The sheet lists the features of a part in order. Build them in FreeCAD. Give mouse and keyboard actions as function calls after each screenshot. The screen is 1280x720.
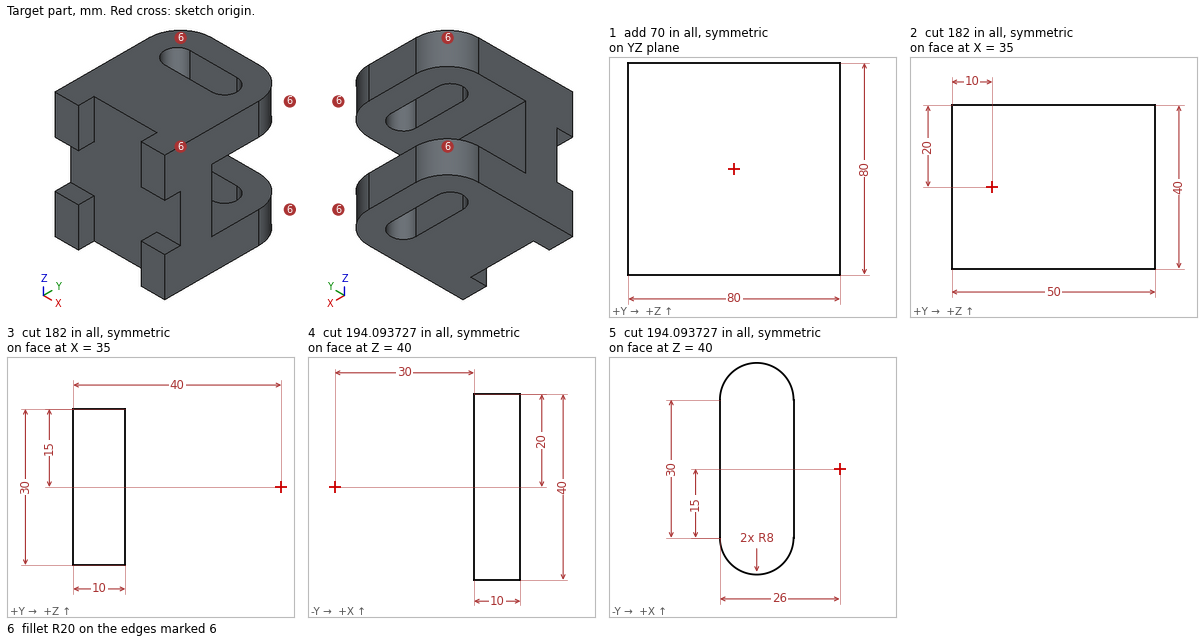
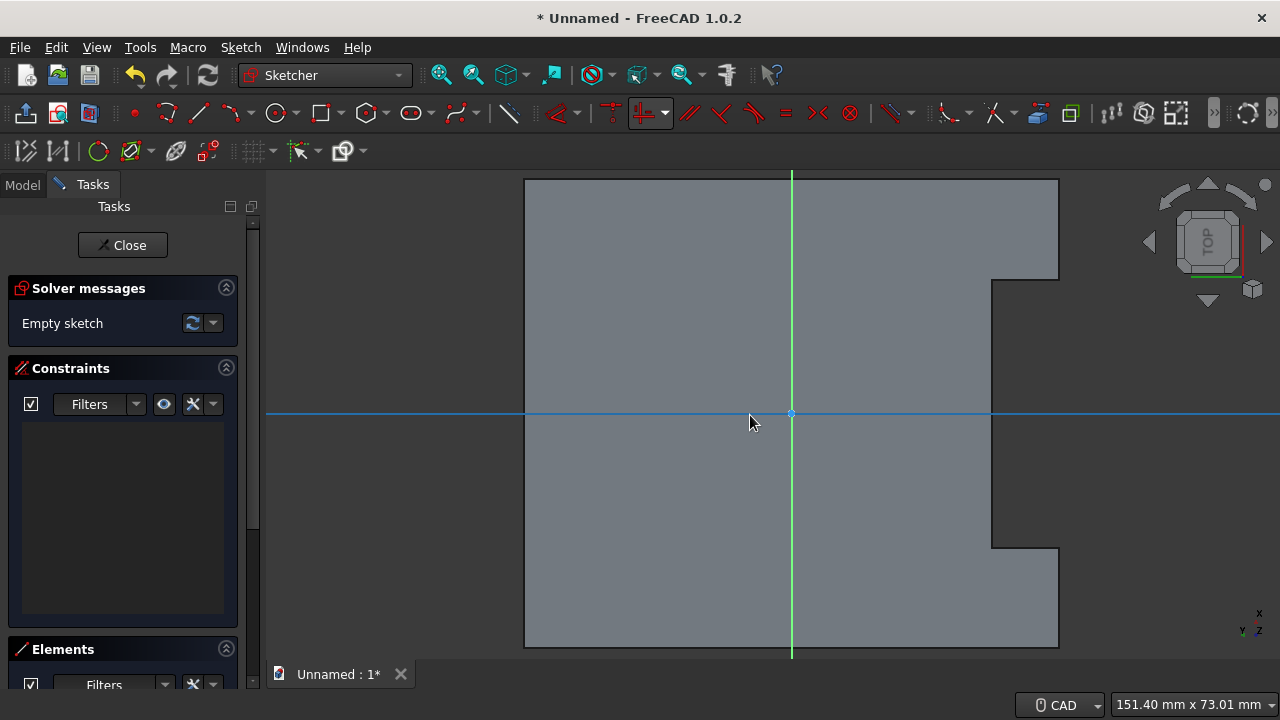
click(412, 114)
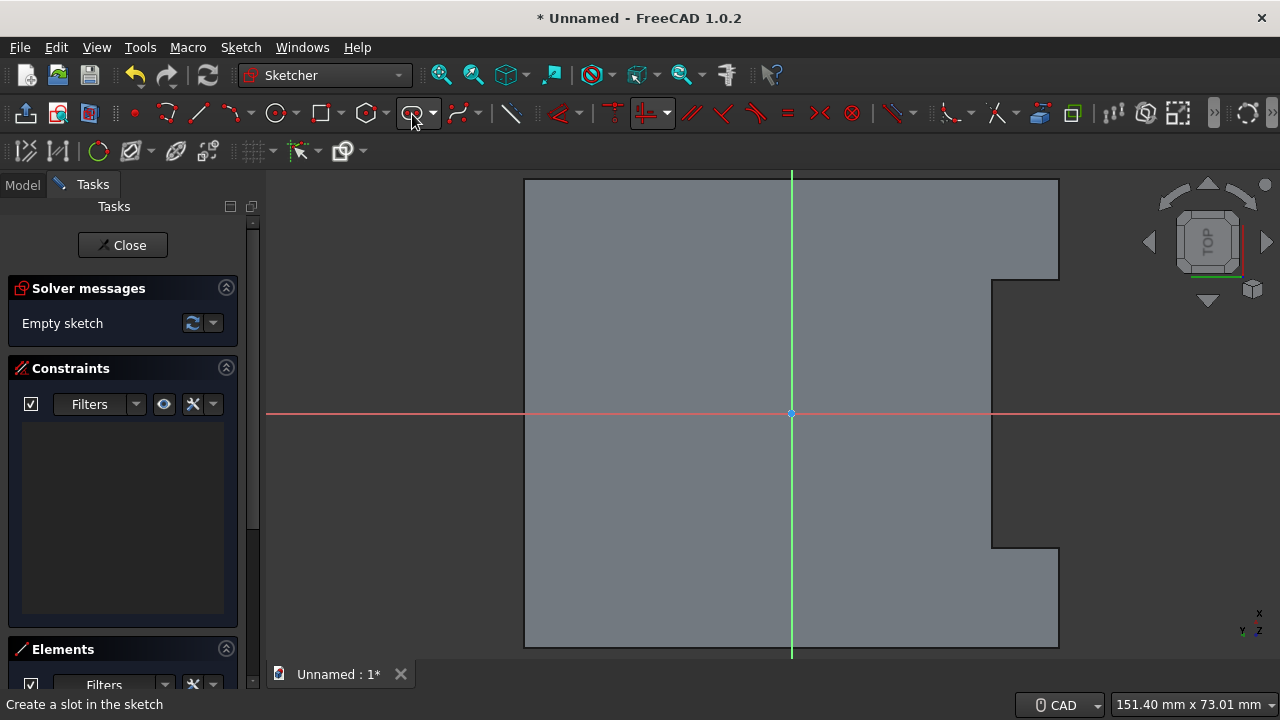
click(671, 514)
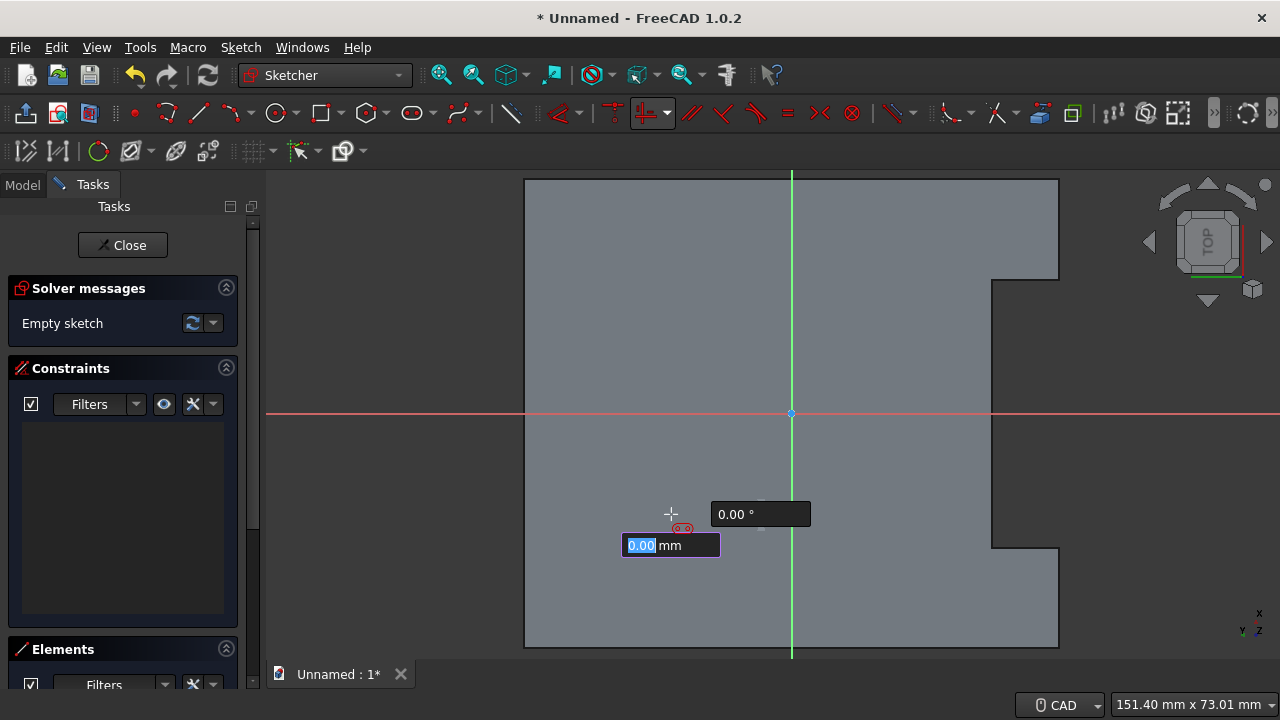
click(671, 313)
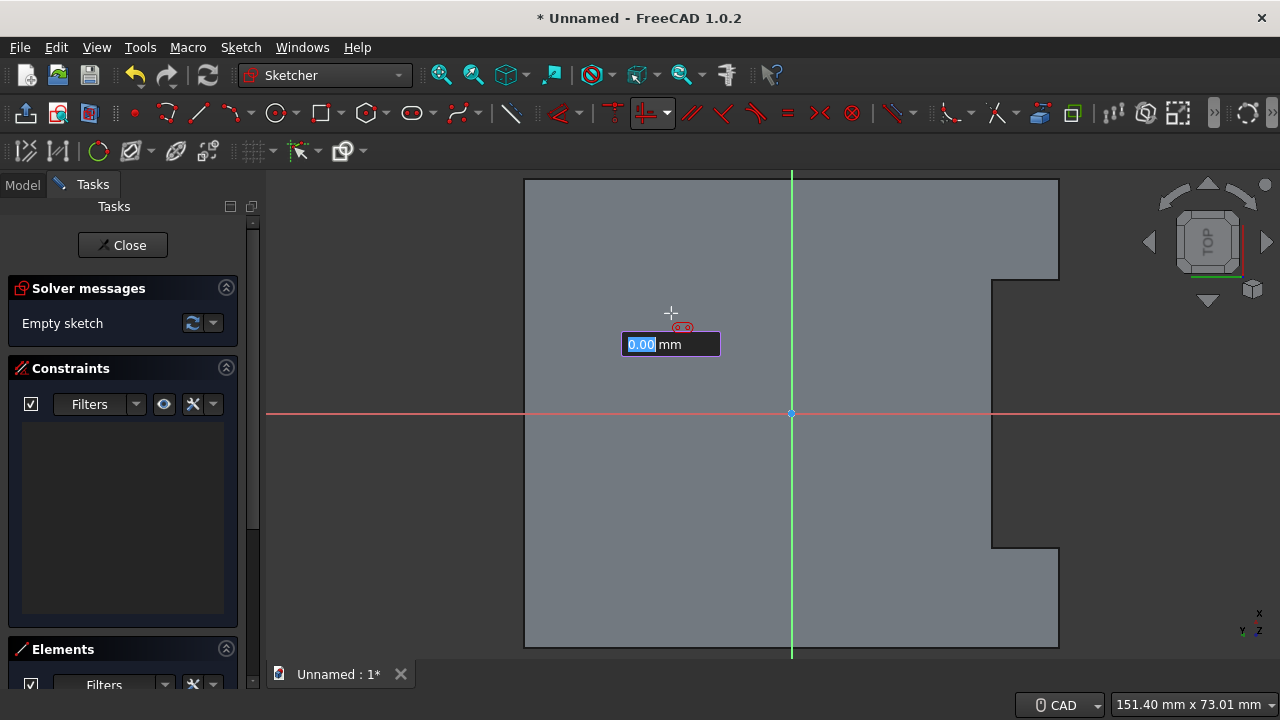
click(617, 384)
key(Escape)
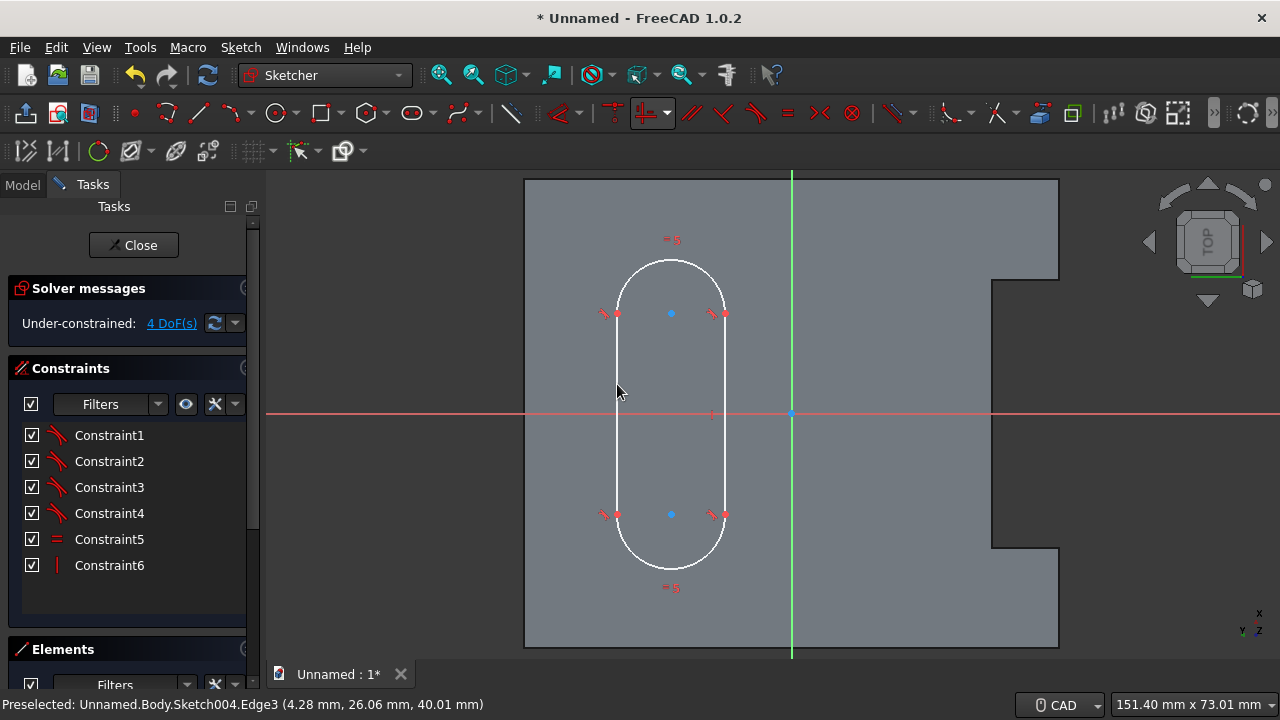
click(558, 114)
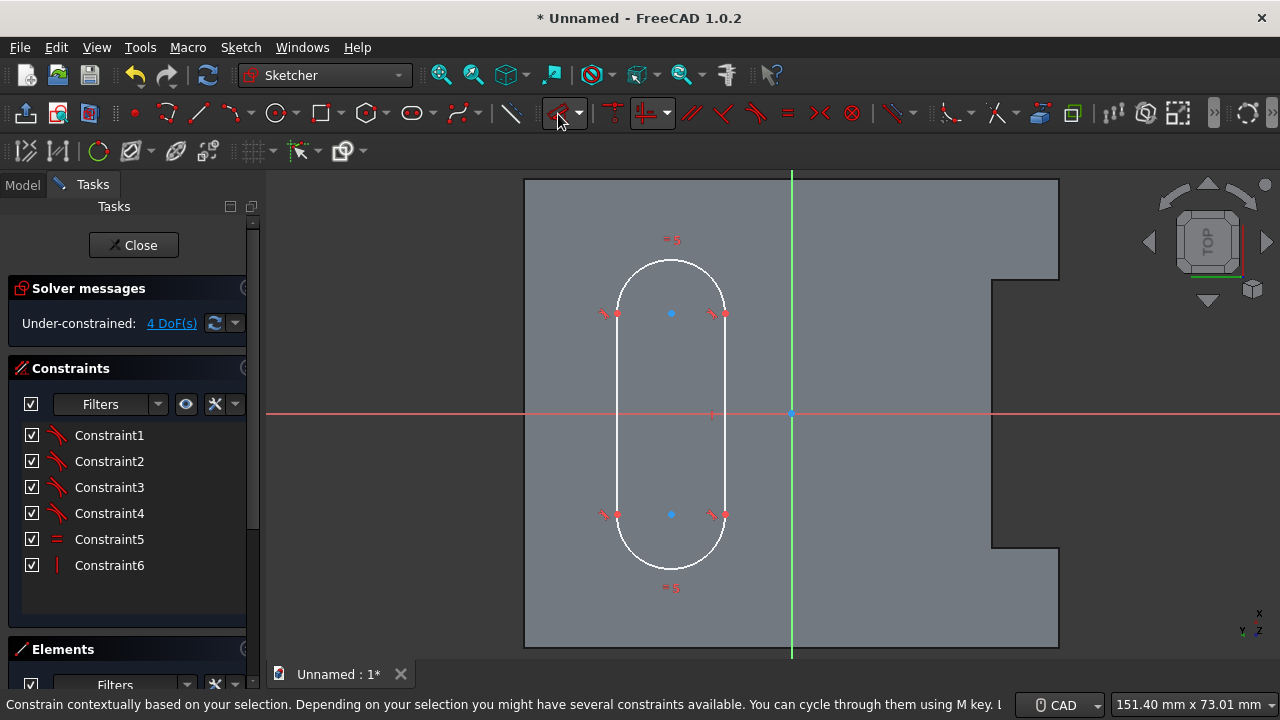
click(639, 559)
click(620, 585)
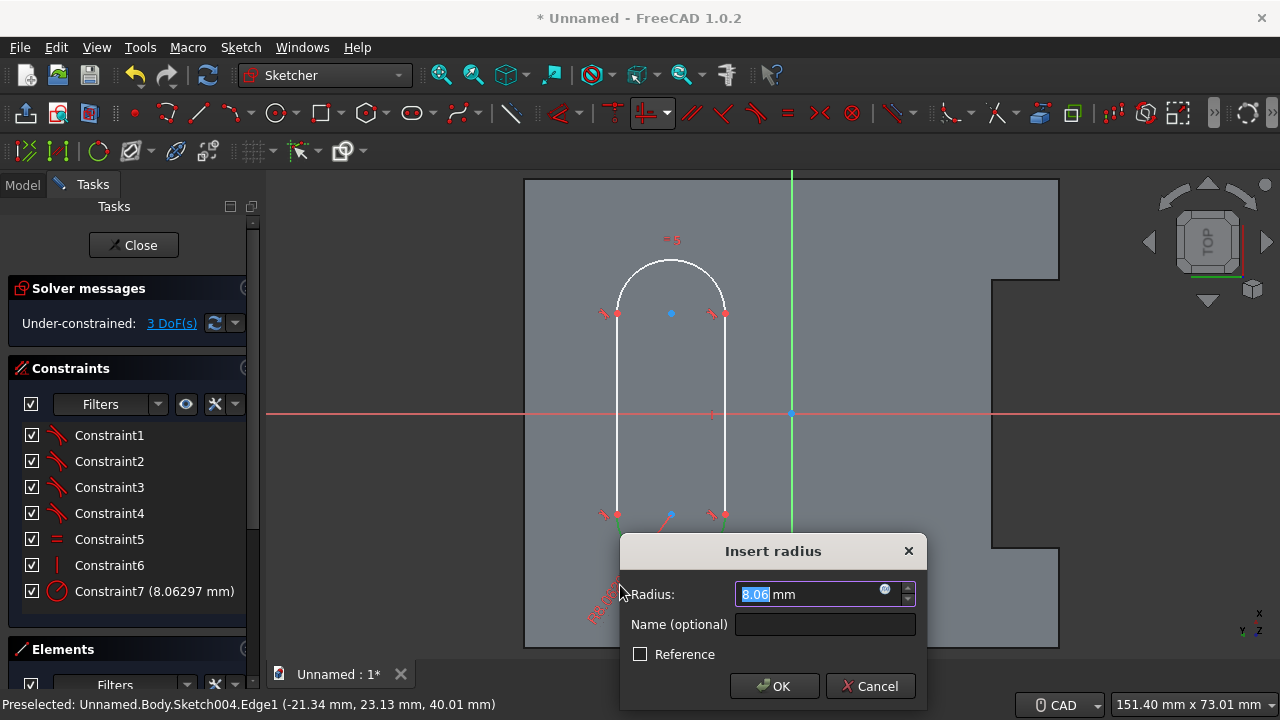
text(8)
key(Return)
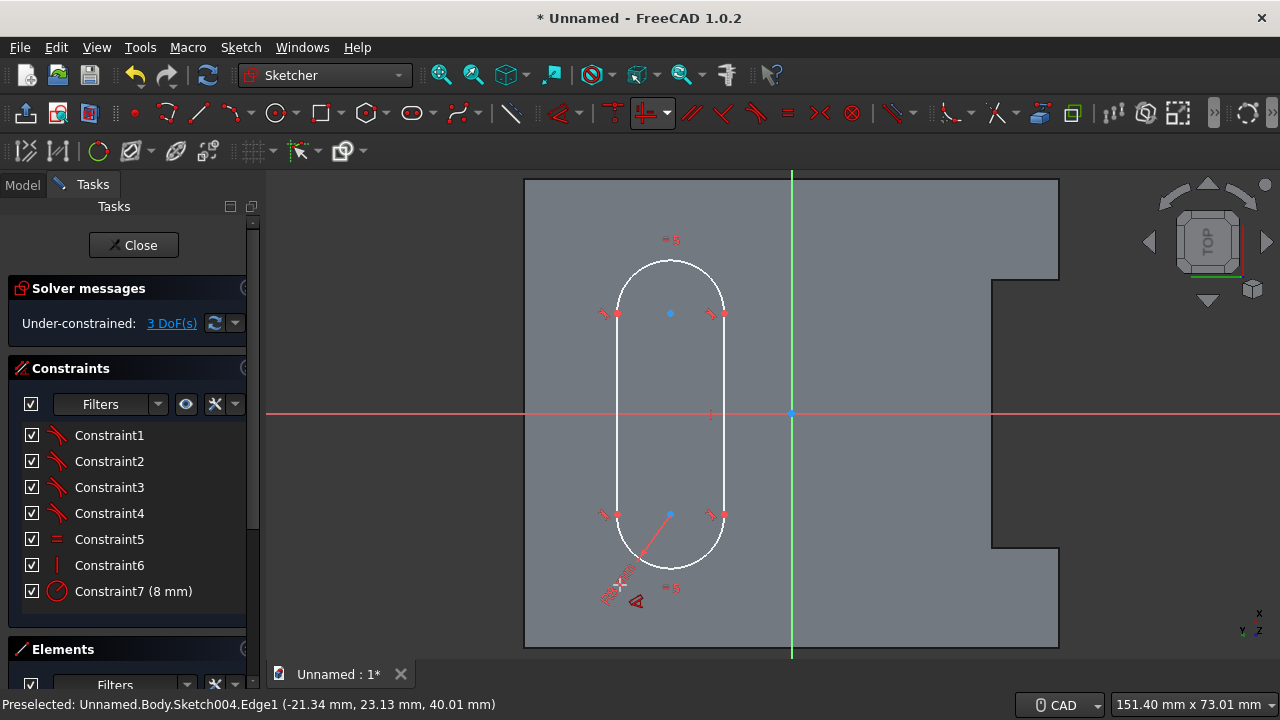
click(617, 455)
click(583, 368)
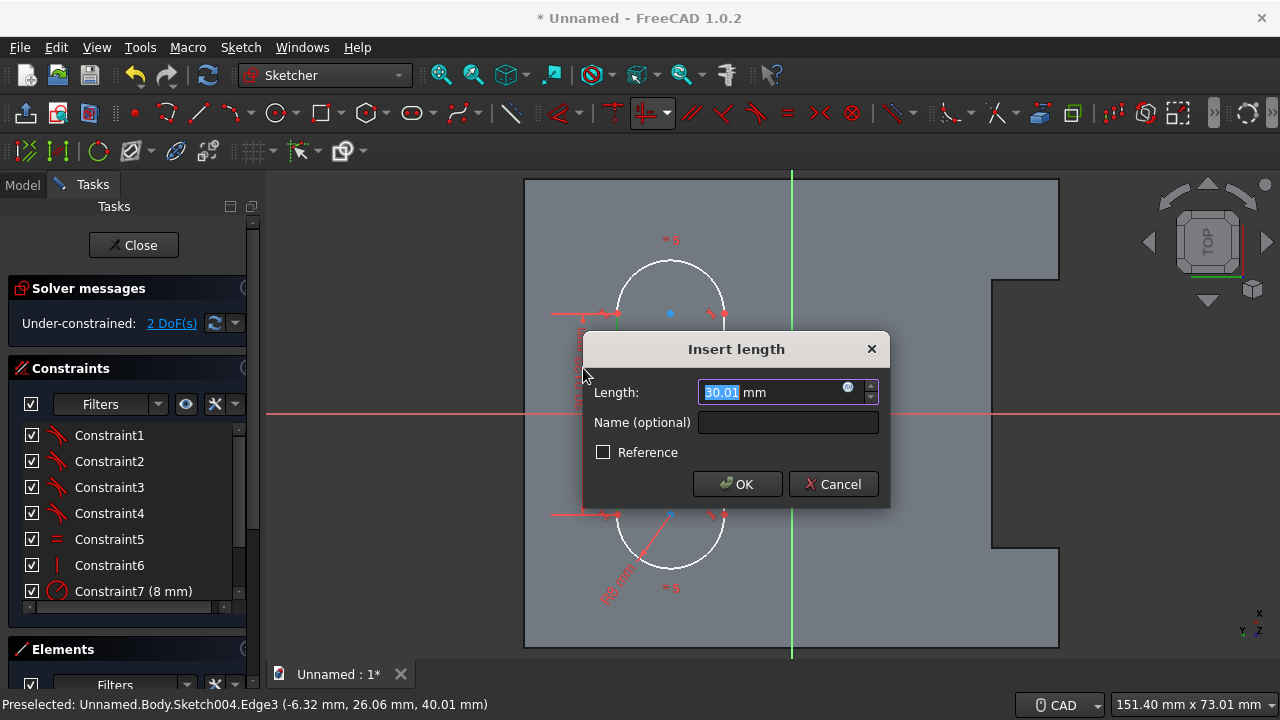
text(30)
key(Return)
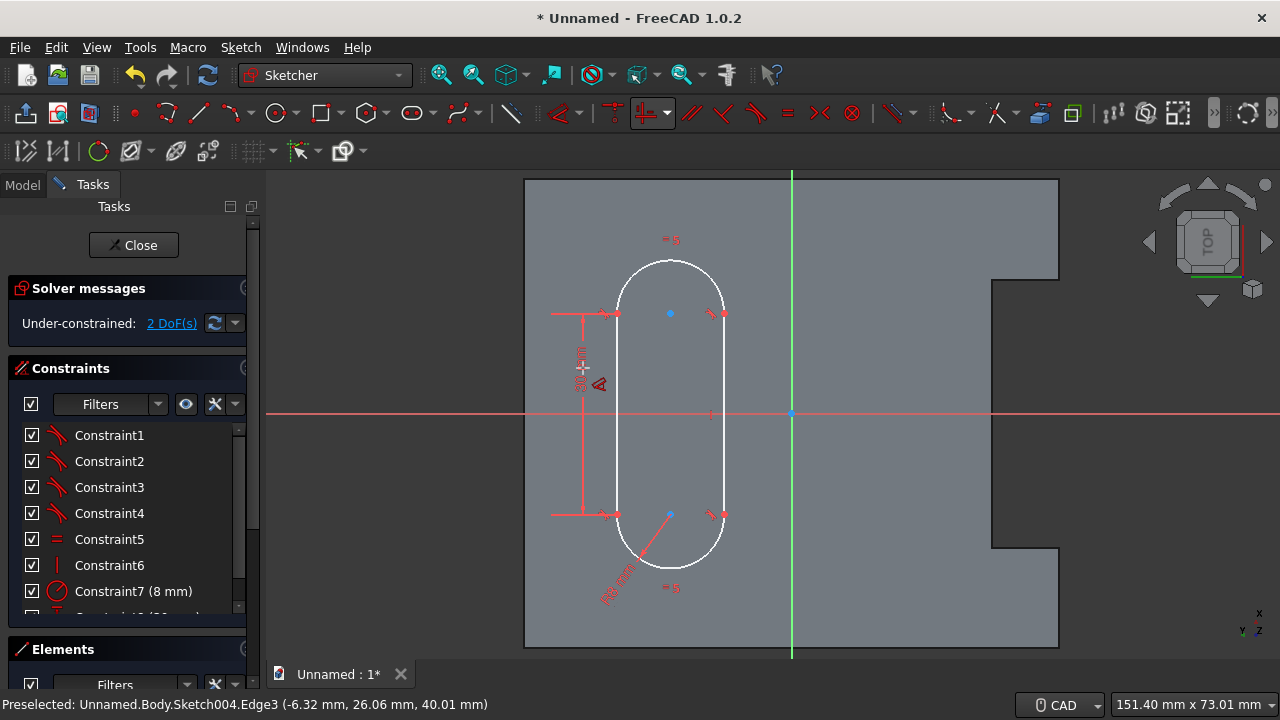
click(617, 515)
click(664, 549)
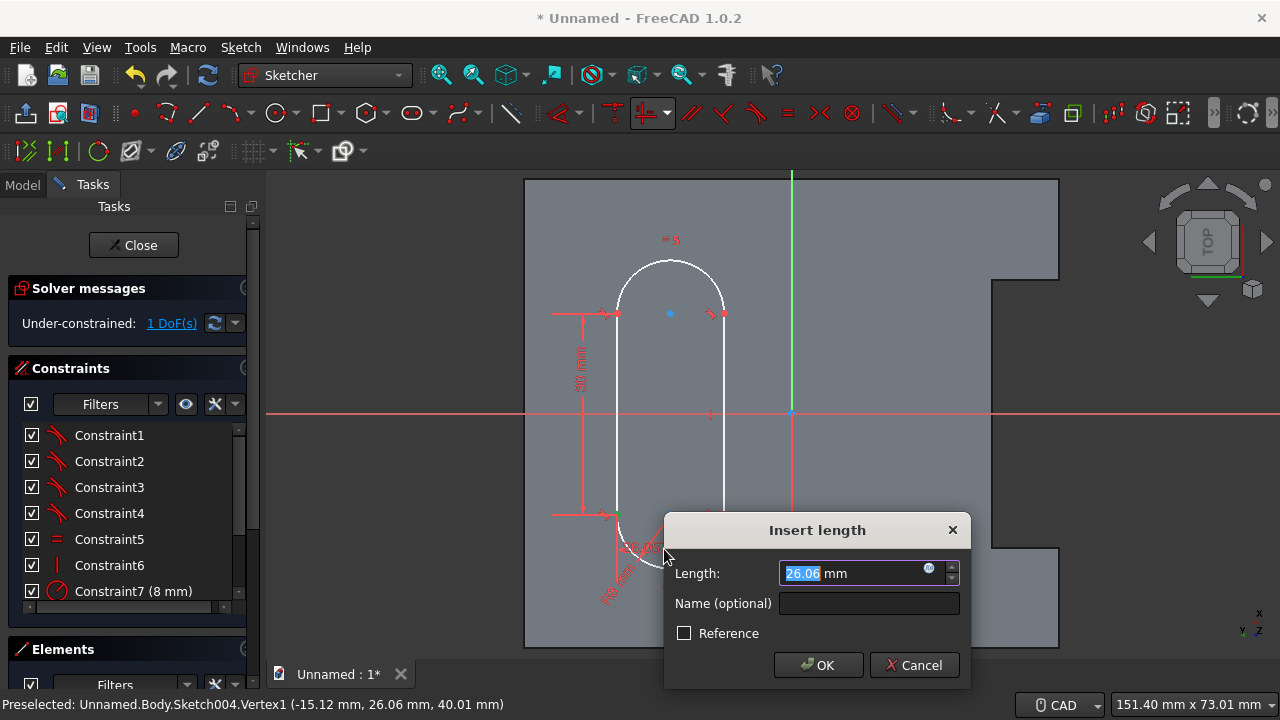
text(26)
key(Return)